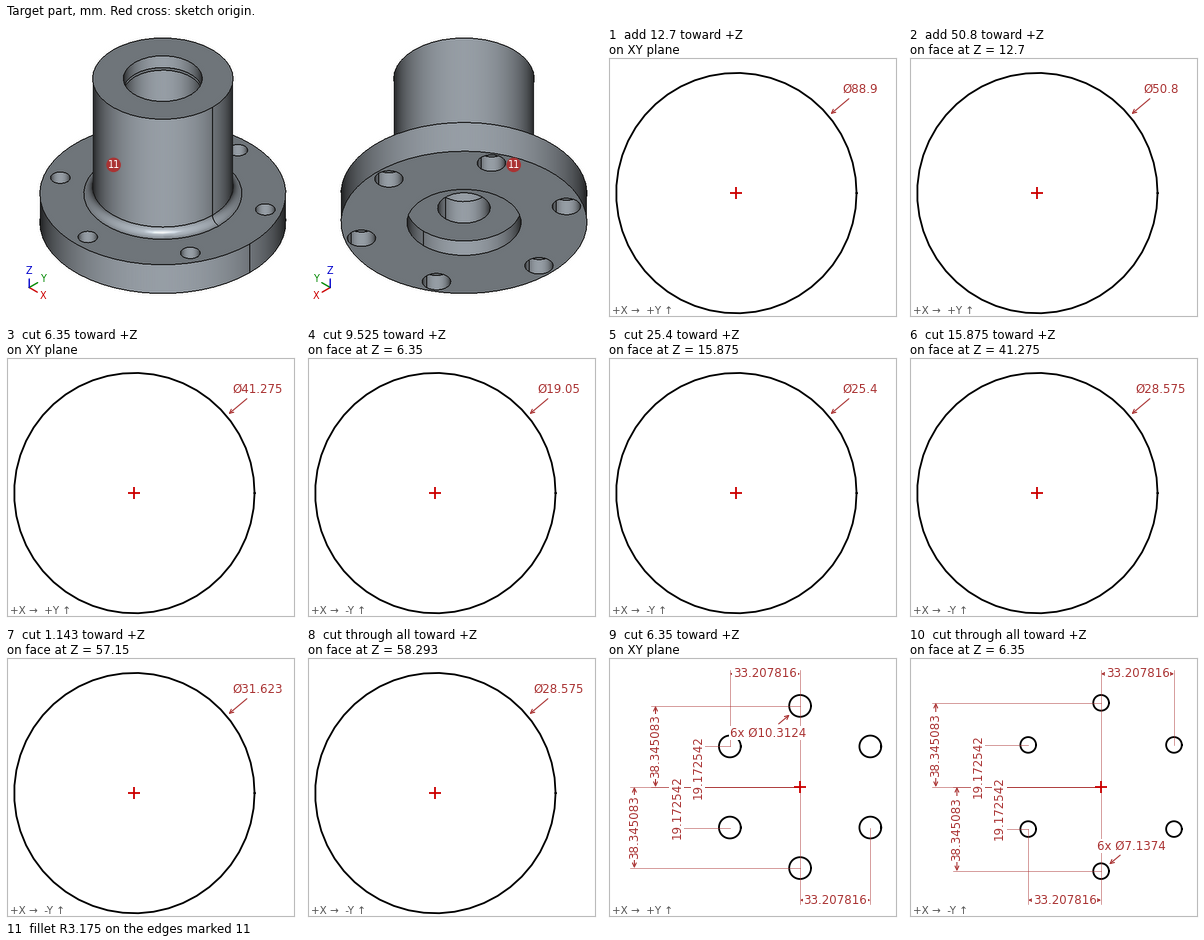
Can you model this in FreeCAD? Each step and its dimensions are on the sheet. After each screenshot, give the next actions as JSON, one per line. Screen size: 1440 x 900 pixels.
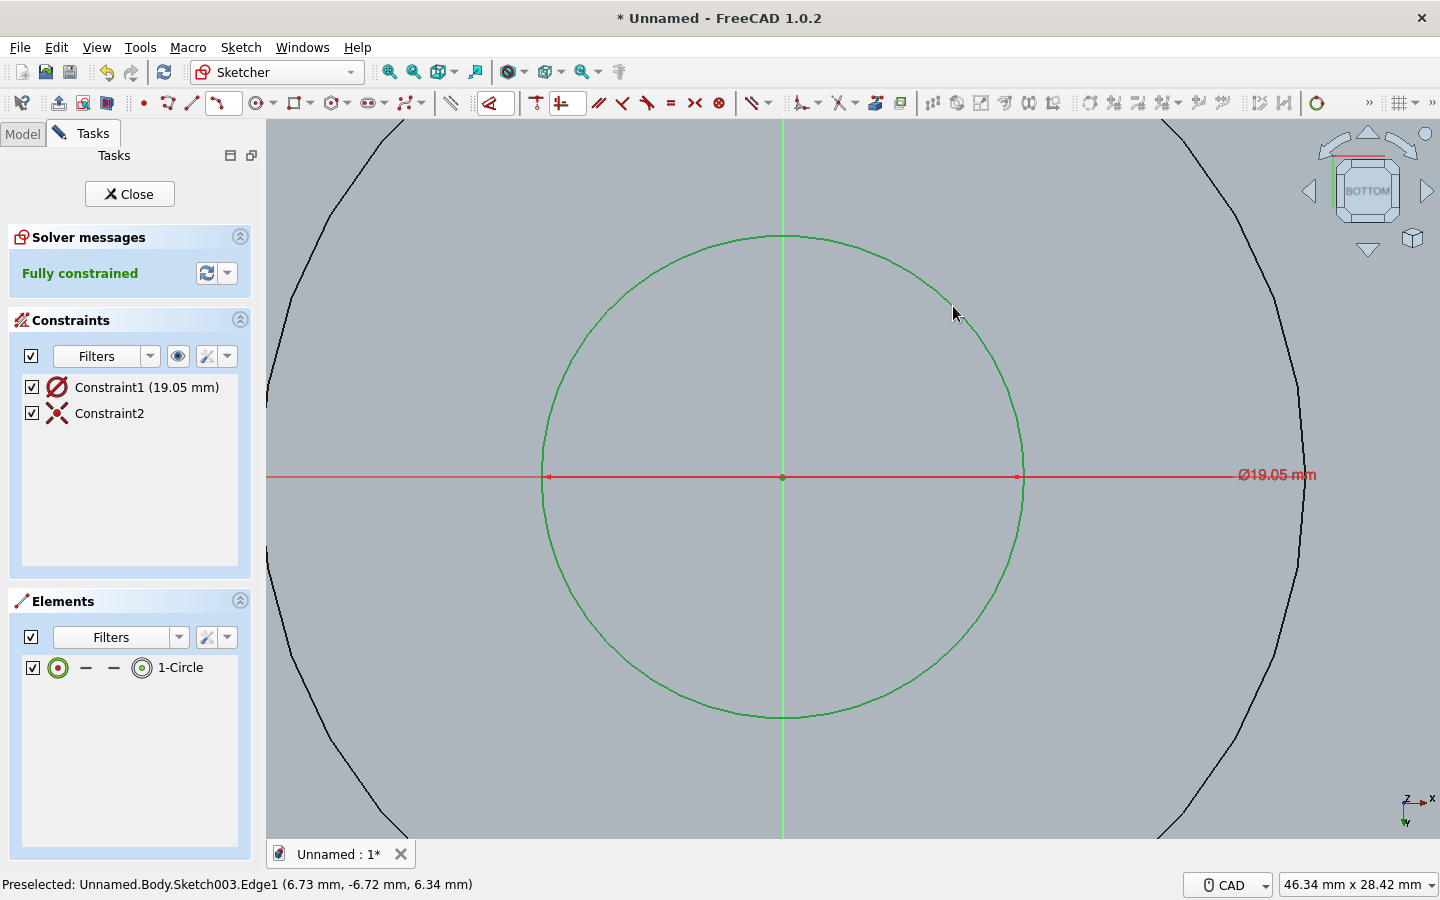
{"action": "left_click", "coordinate": [130, 194]}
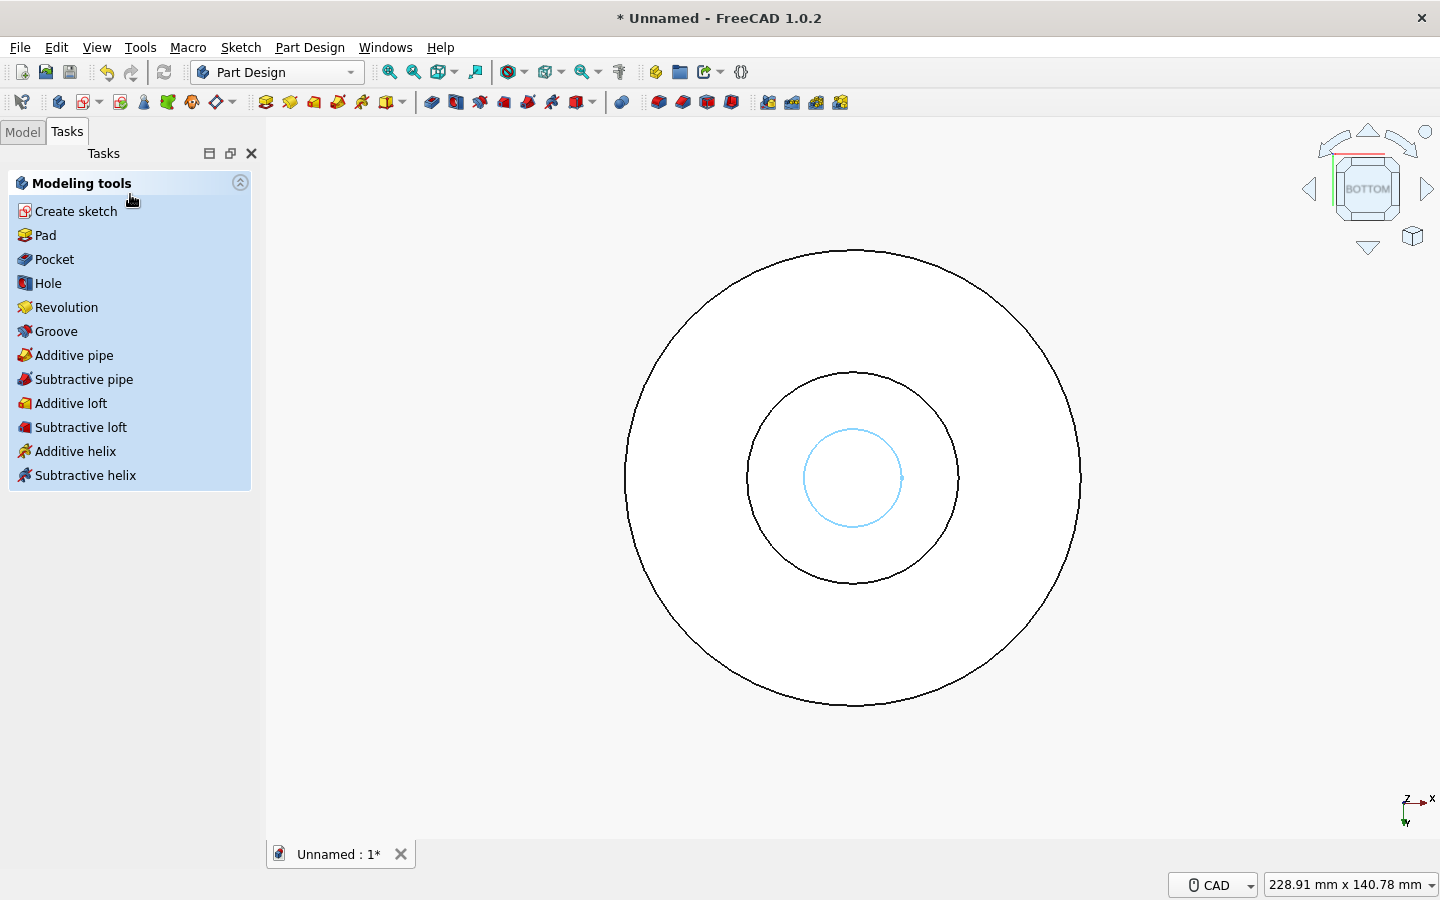
{"action": "left_click", "coordinate": [432, 102]}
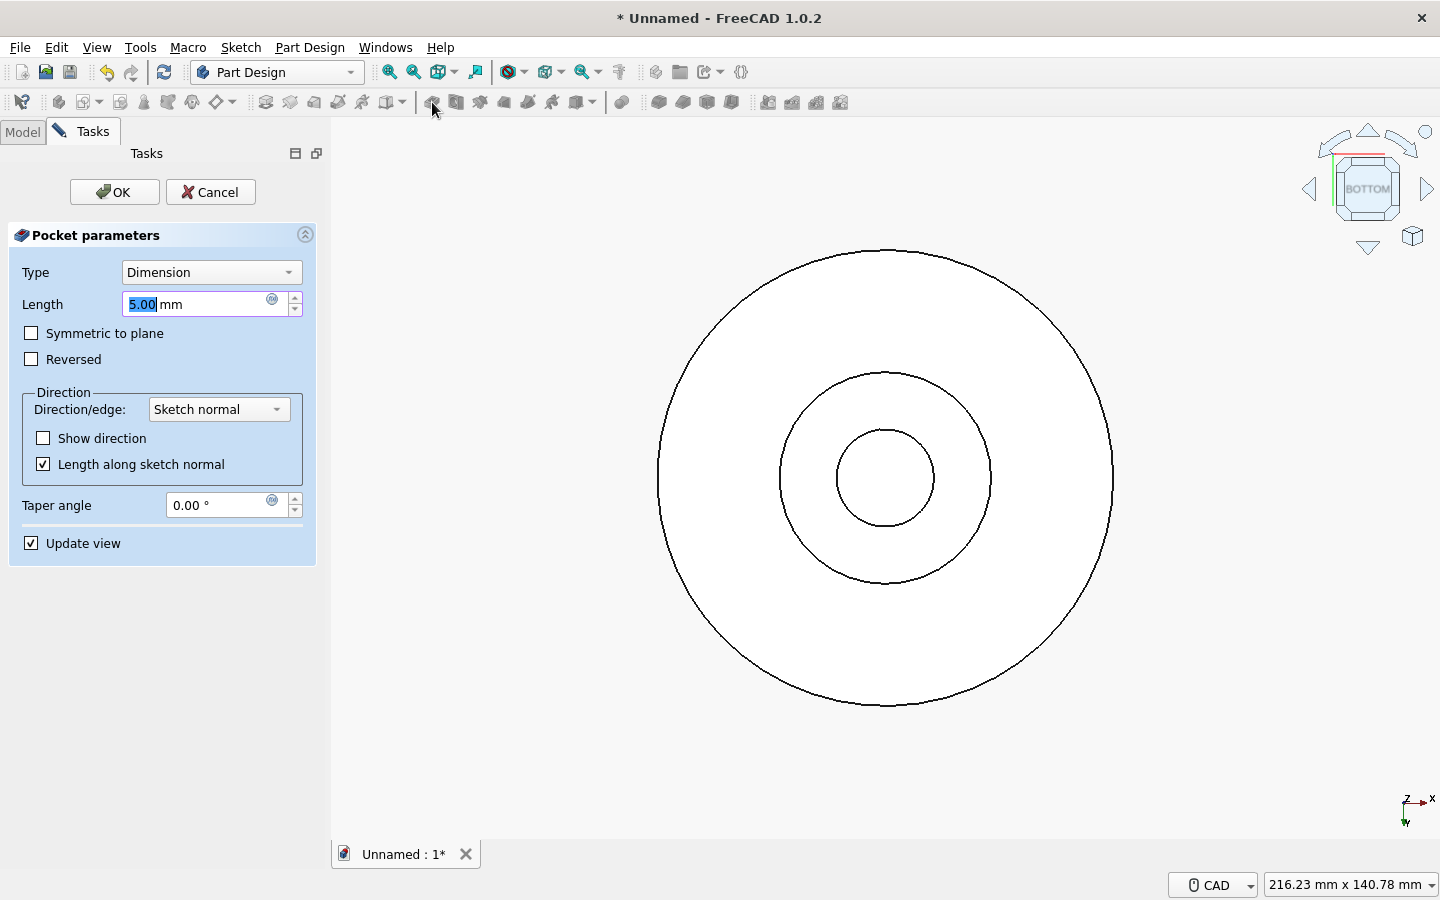
{"action": "type", "text": "9.525"}
{"action": "key", "text": "Tab"}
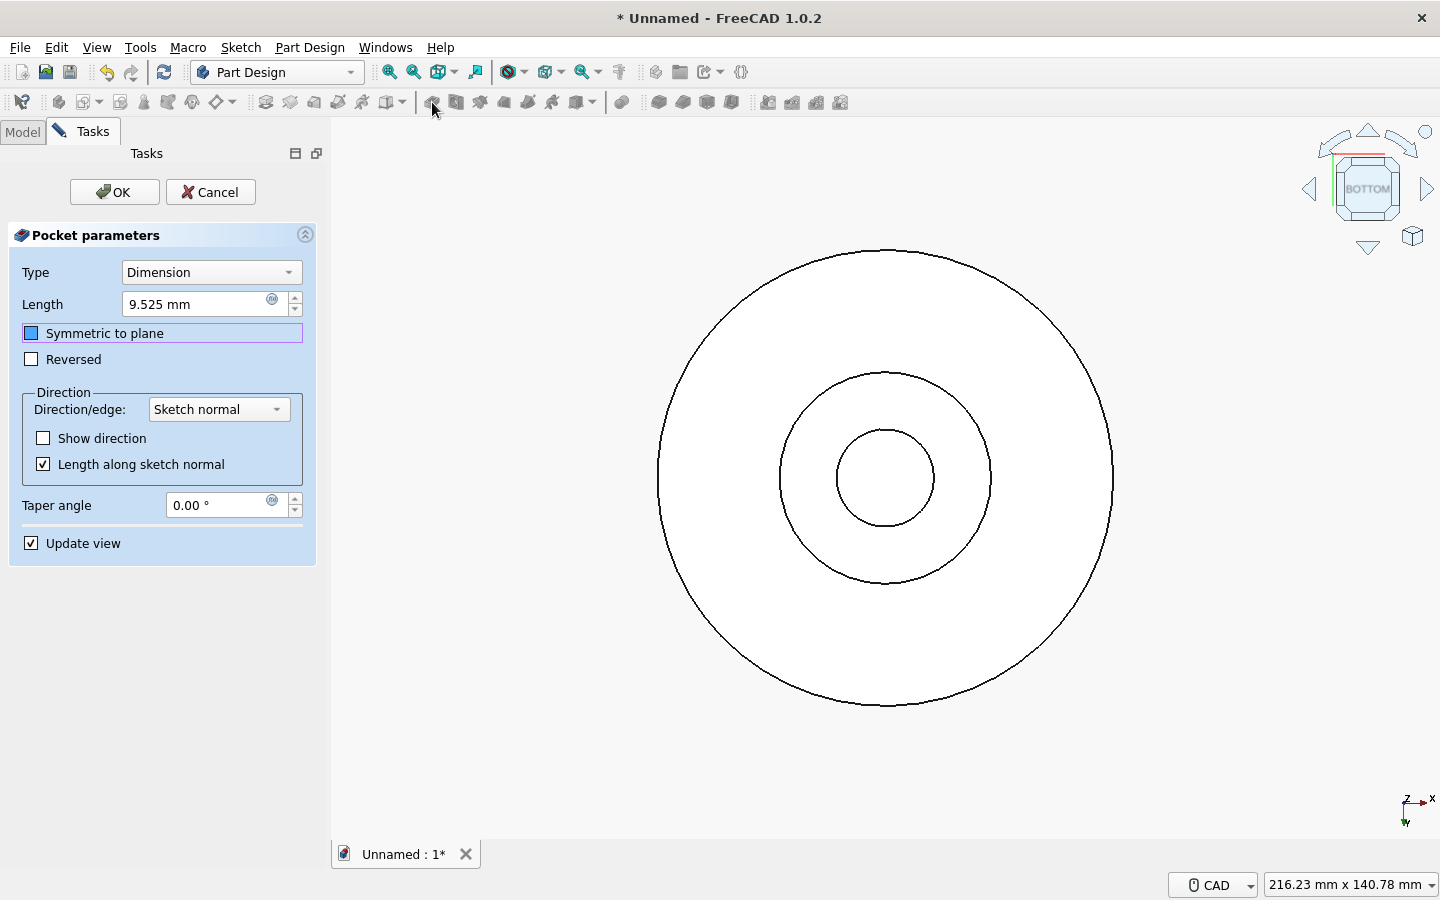
{"action": "left_click", "coordinate": [115, 192]}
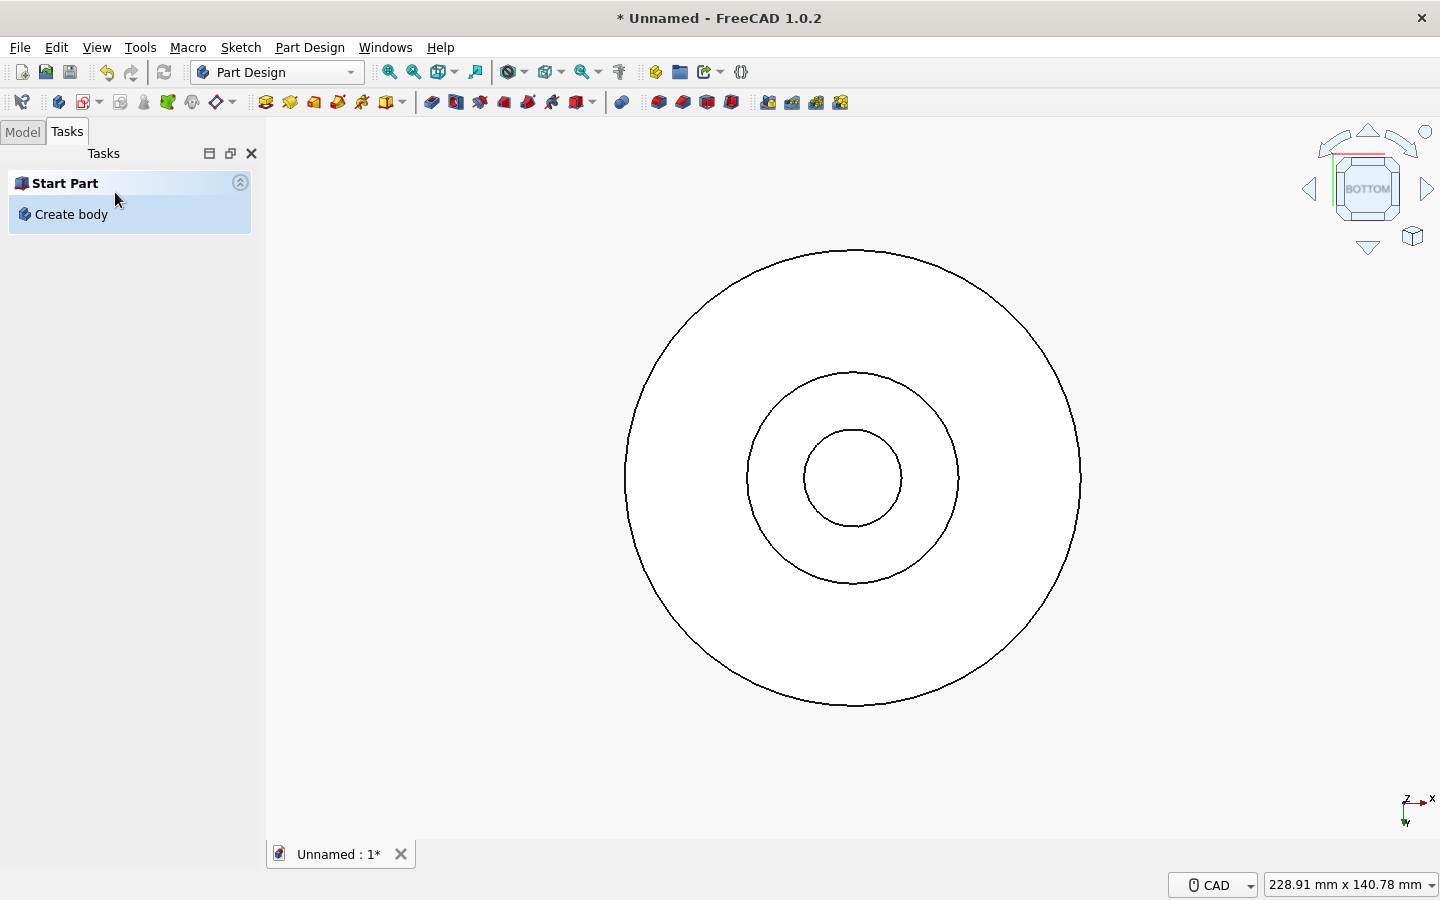
{"action": "left_click", "coordinate": [853, 477]}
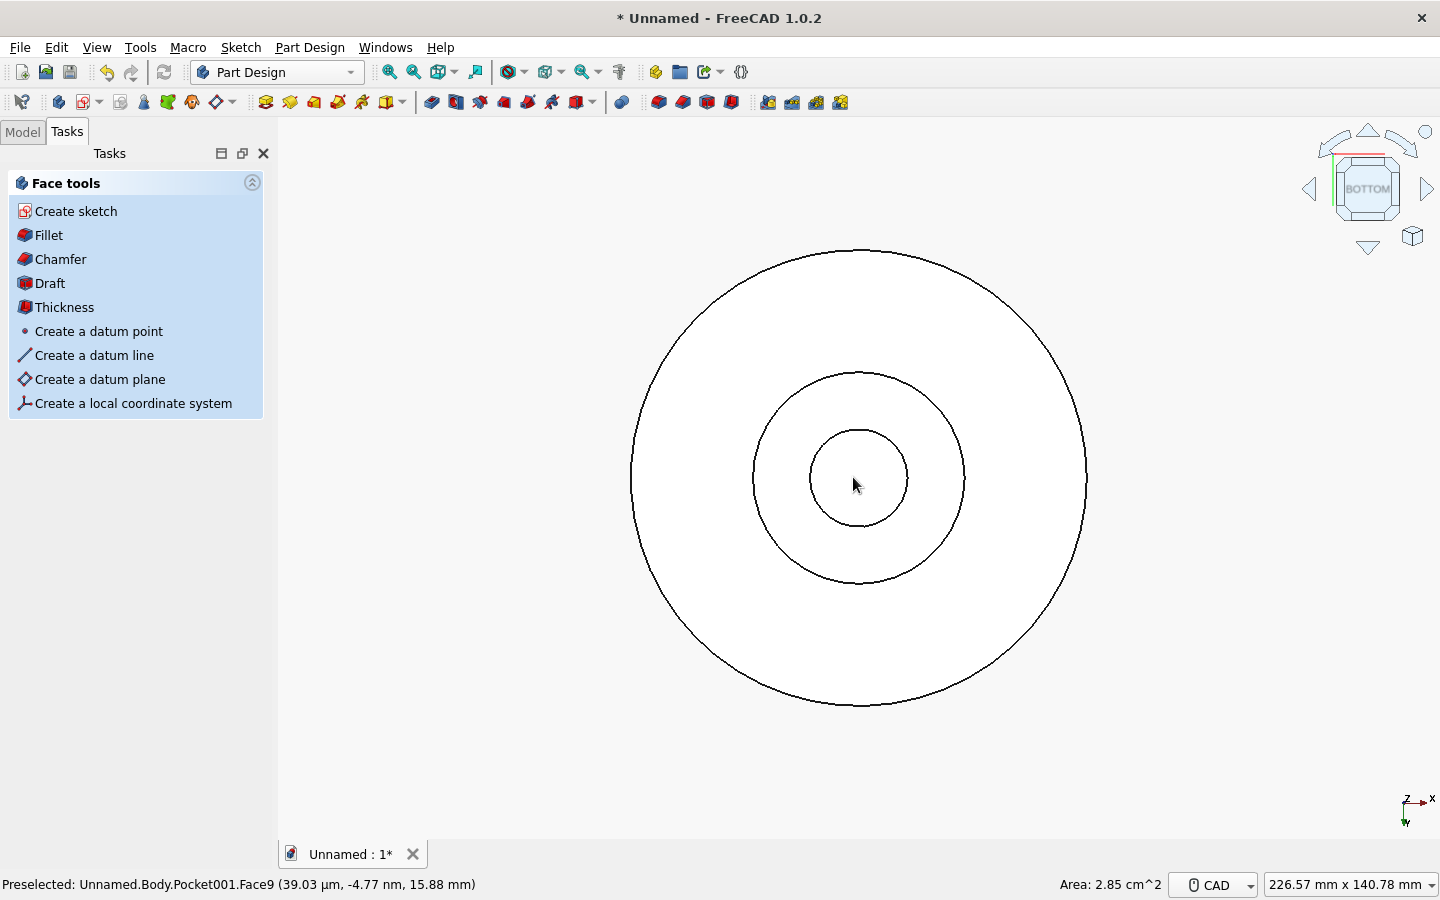
{"action": "left_click", "coordinate": [84, 102]}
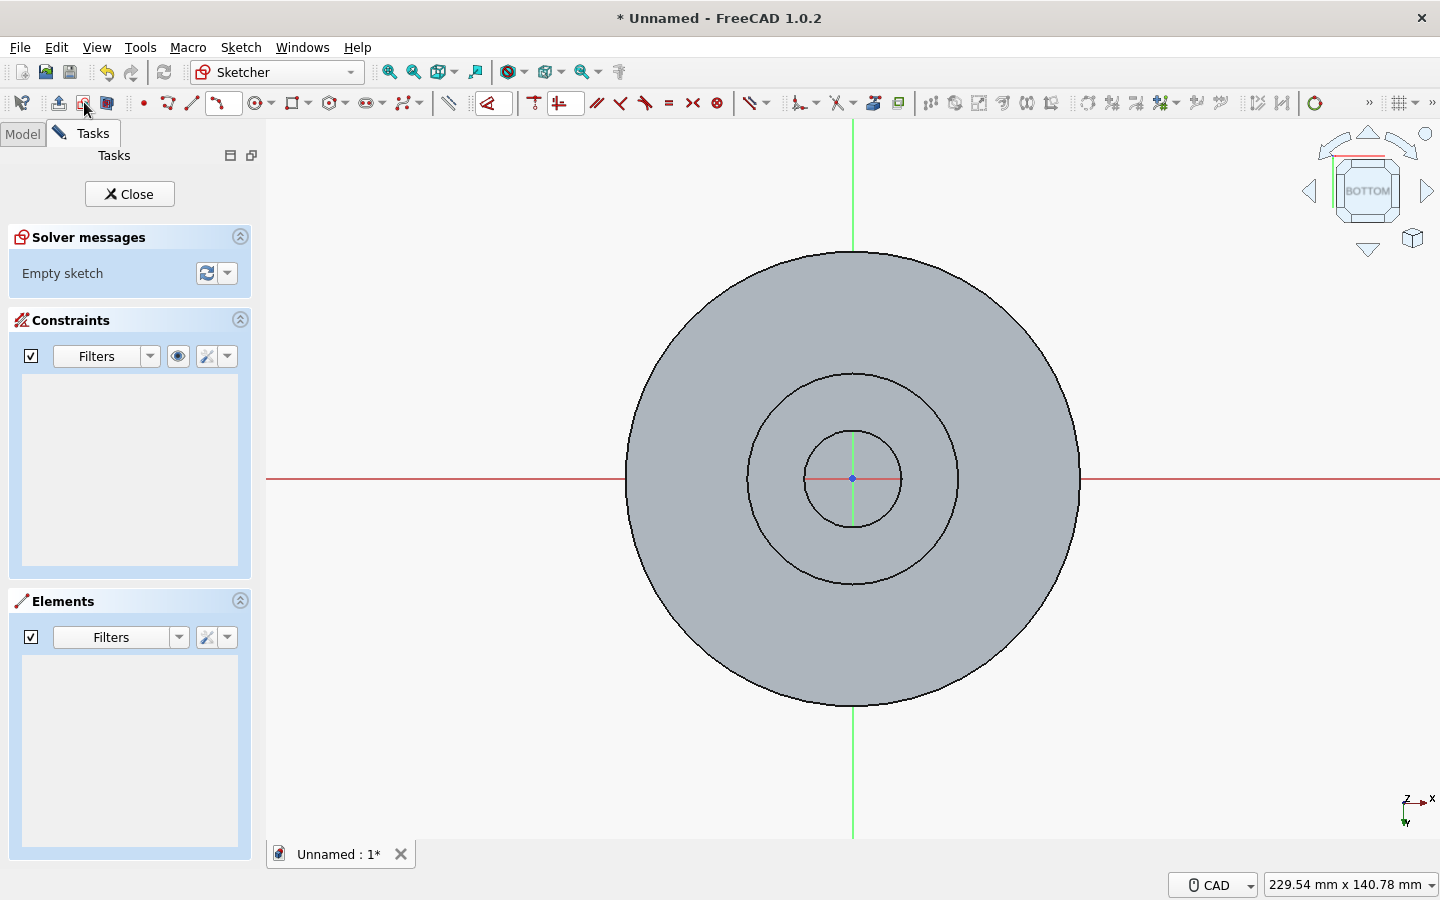
{"action": "scroll", "coordinate": [882, 479], "scroll_direction": "up", "scroll_amount": 6}